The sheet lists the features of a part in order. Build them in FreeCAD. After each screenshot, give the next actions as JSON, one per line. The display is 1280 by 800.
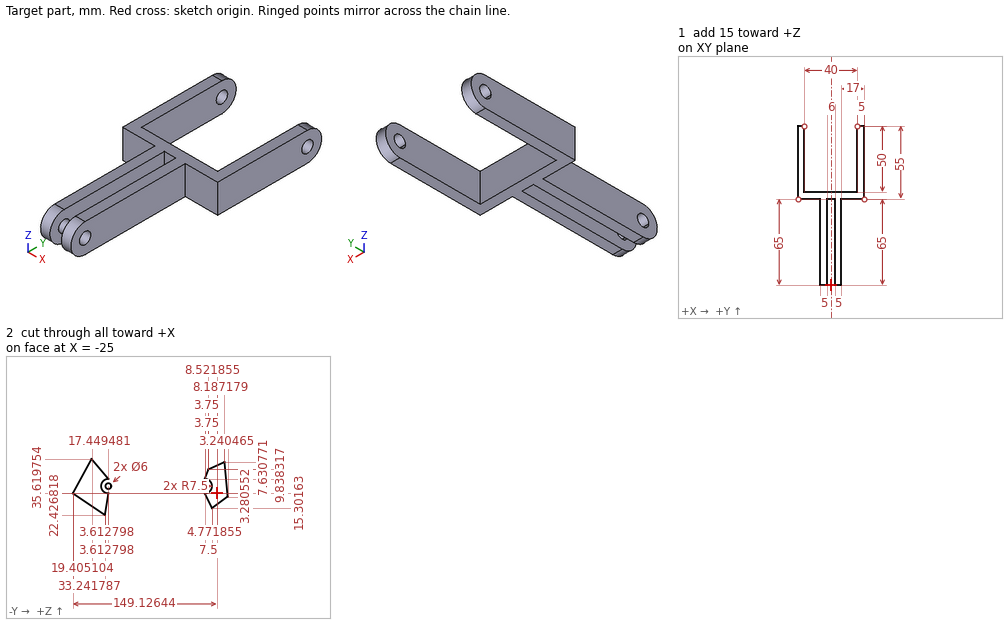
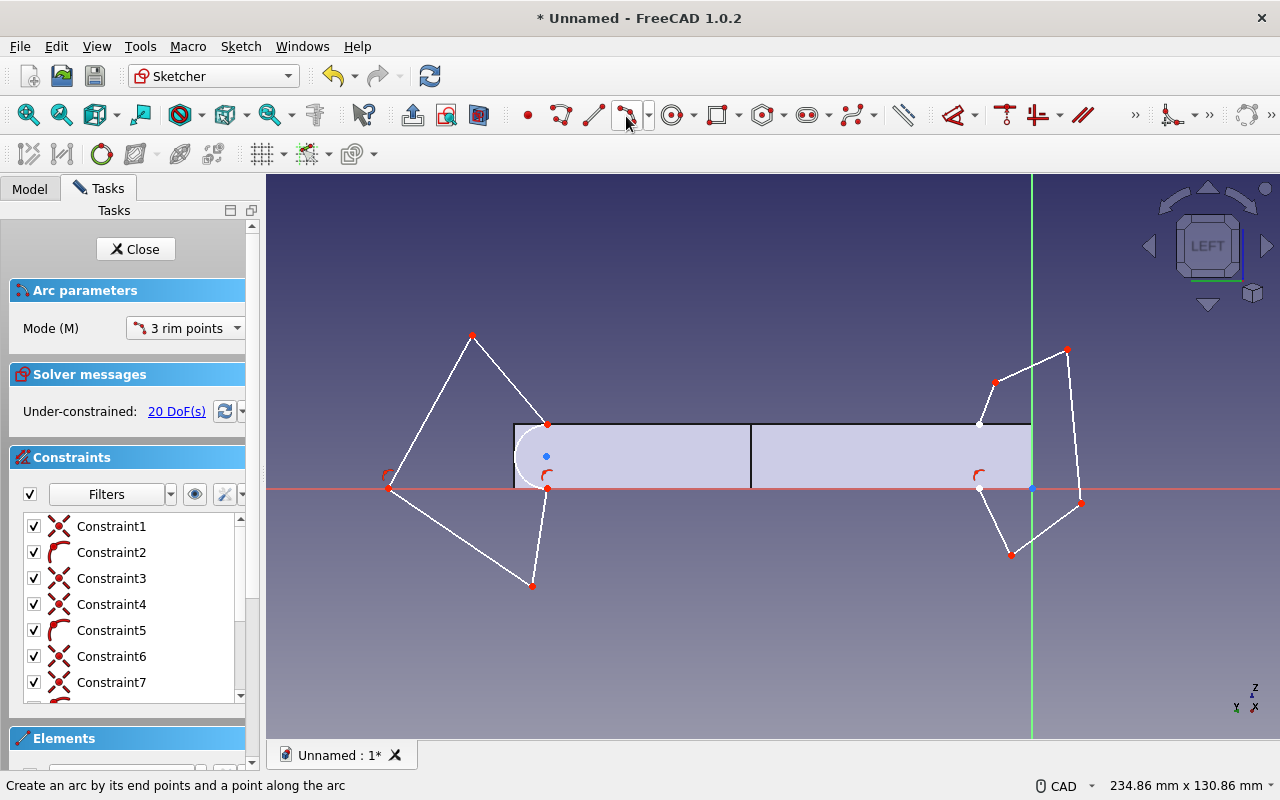
{"action": "left_click", "coordinate": [979, 425]}
{"action": "left_click", "coordinate": [979, 489]}
{"action": "left_click", "coordinate": [1011, 456]}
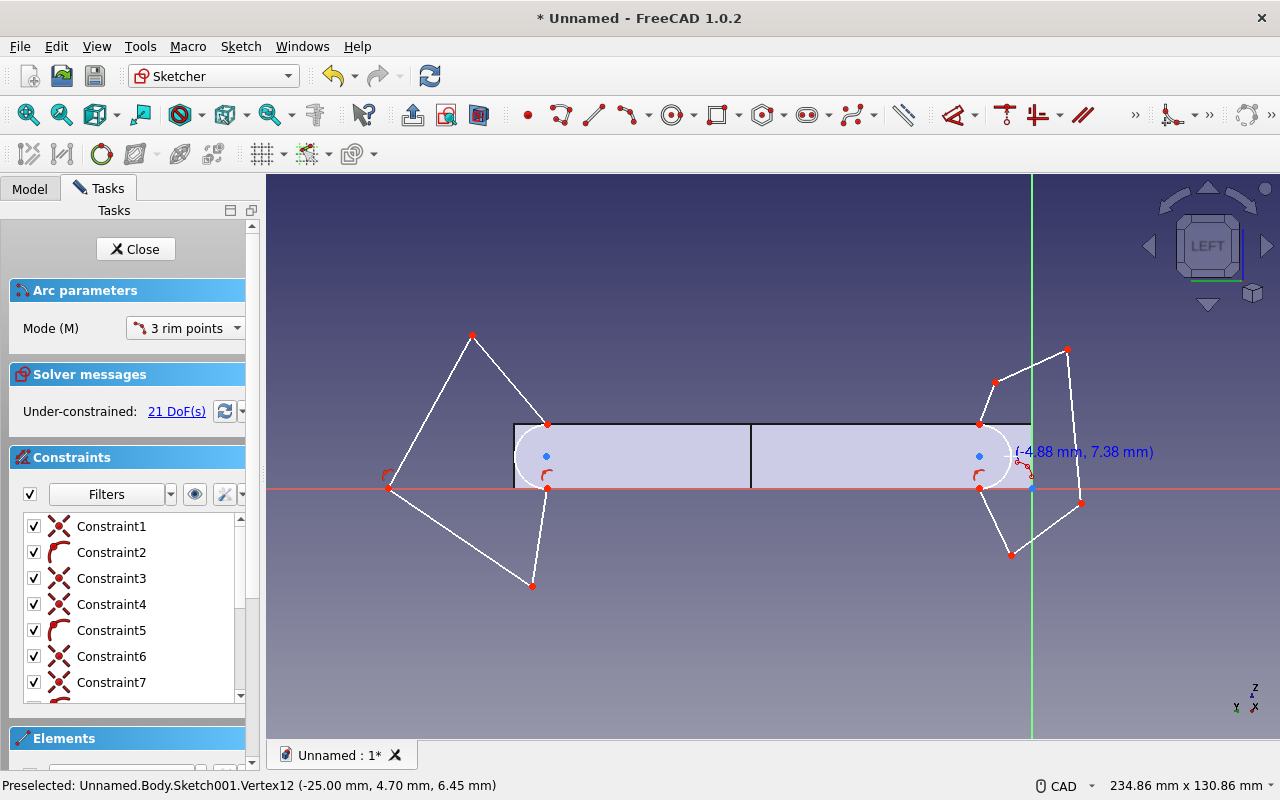
{"action": "key", "text": "g c"}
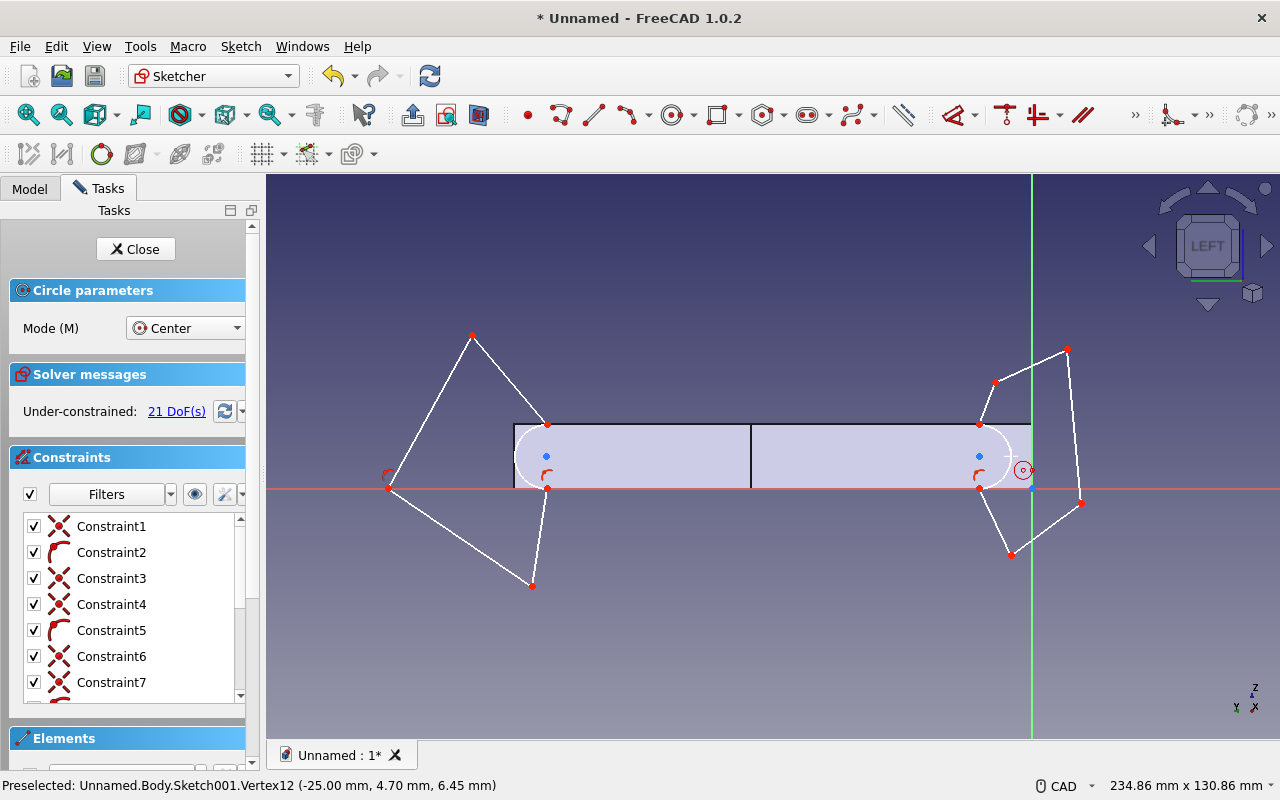
{"action": "scroll", "coordinate": [547, 456], "scroll_direction": "up", "scroll_amount": 3}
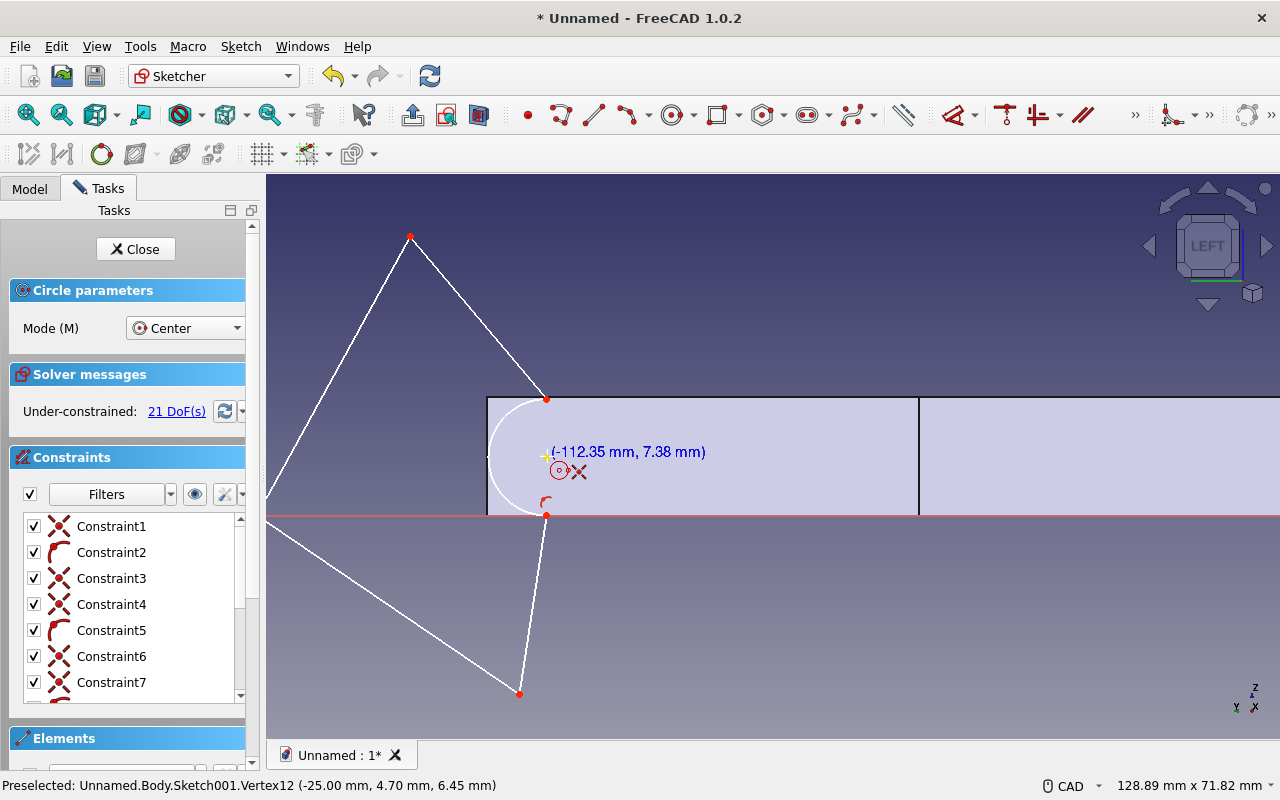
{"action": "left_click", "coordinate": [547, 456]}
{"action": "mouse_move", "coordinate": [564, 440]}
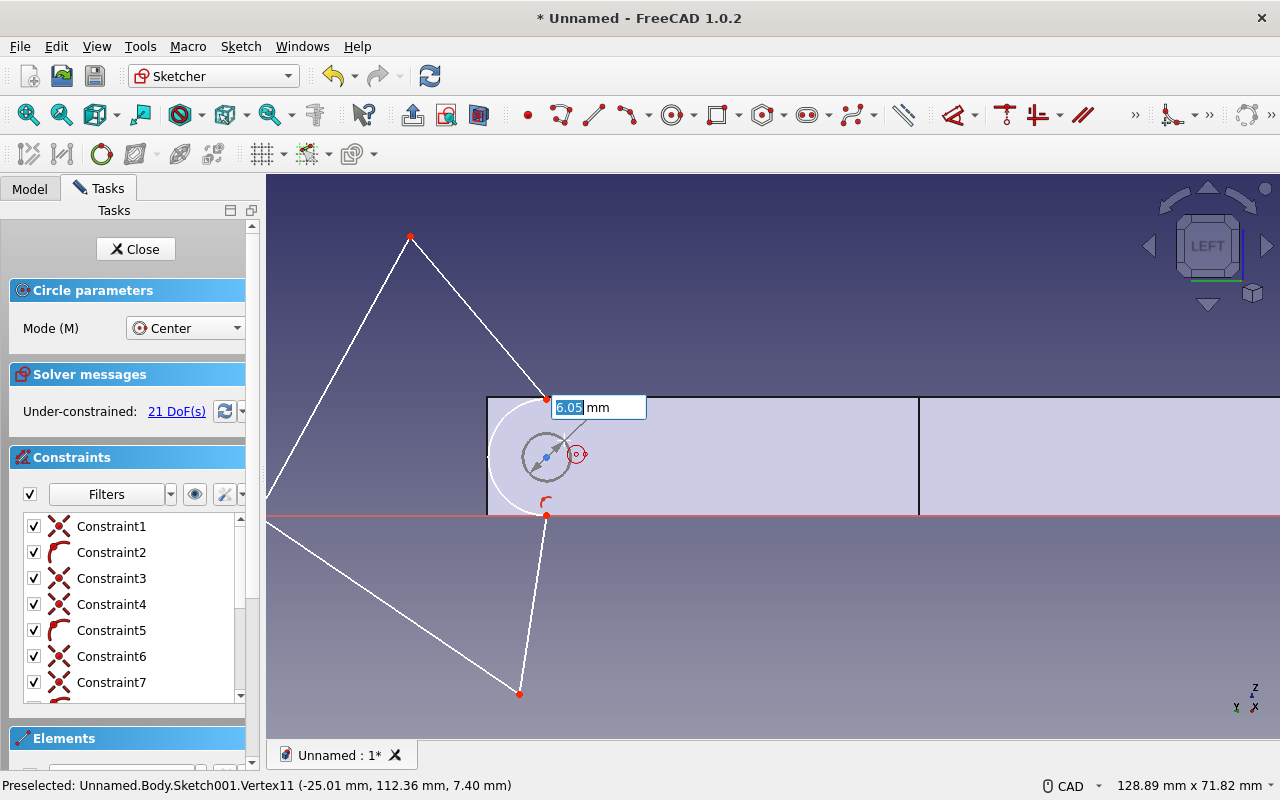
{"action": "type", "text": "6"}
{"action": "key", "text": "Return"}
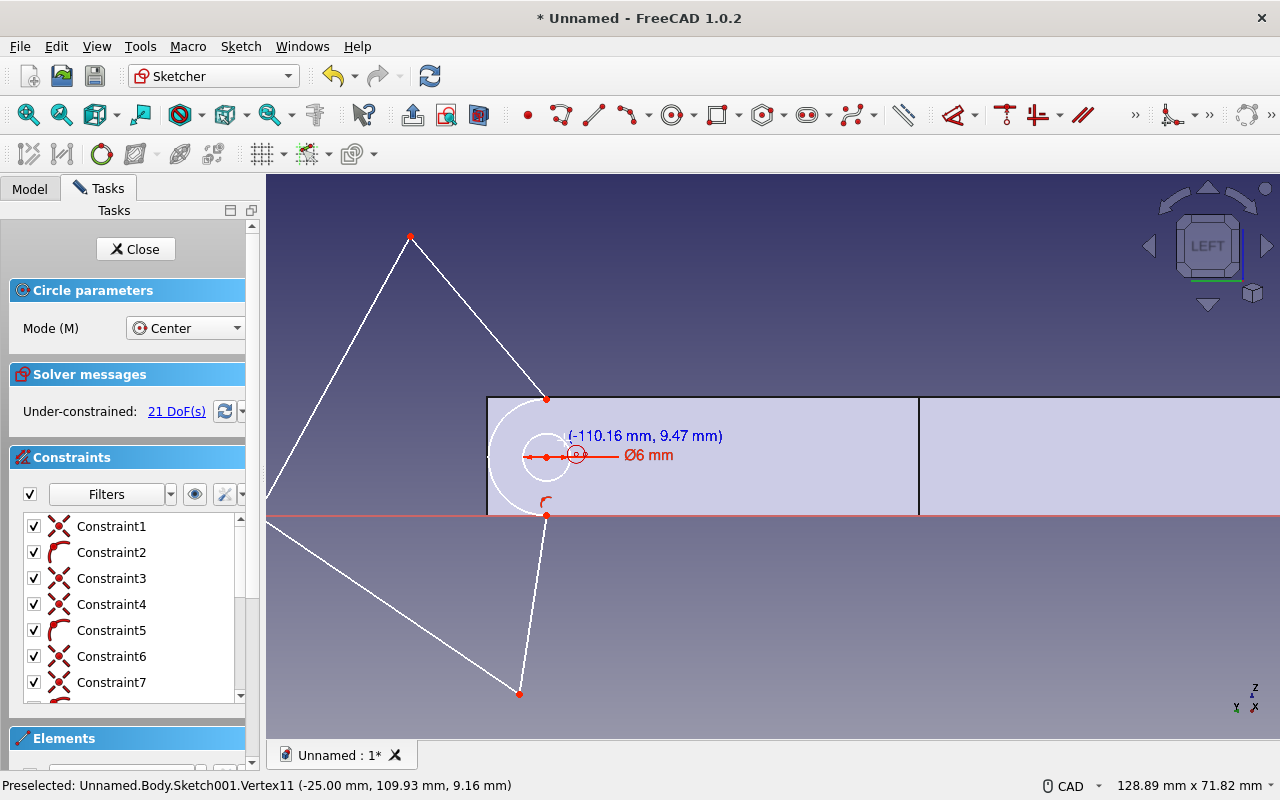
{"action": "scroll", "coordinate": [554, 451], "scroll_direction": "down", "scroll_amount": 4}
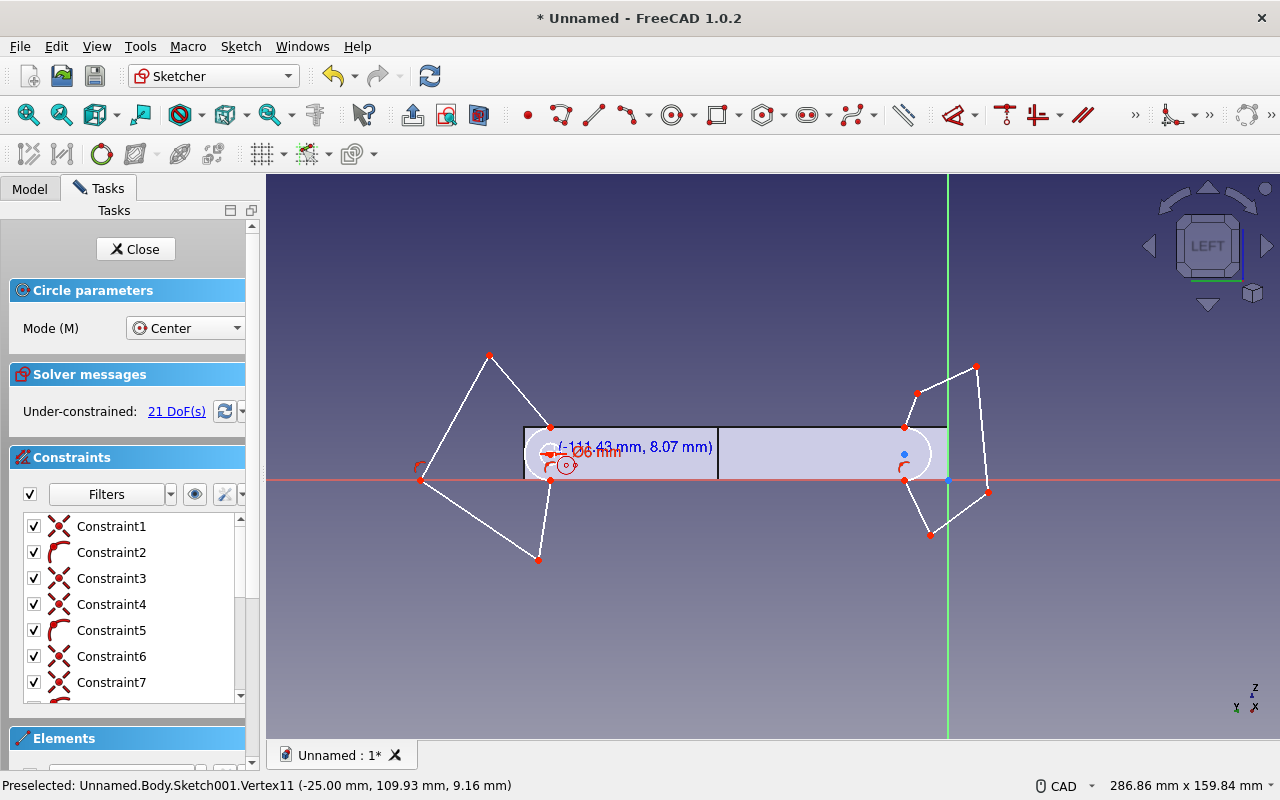
{"action": "scroll", "coordinate": [905, 454], "scroll_direction": "up", "scroll_amount": 4}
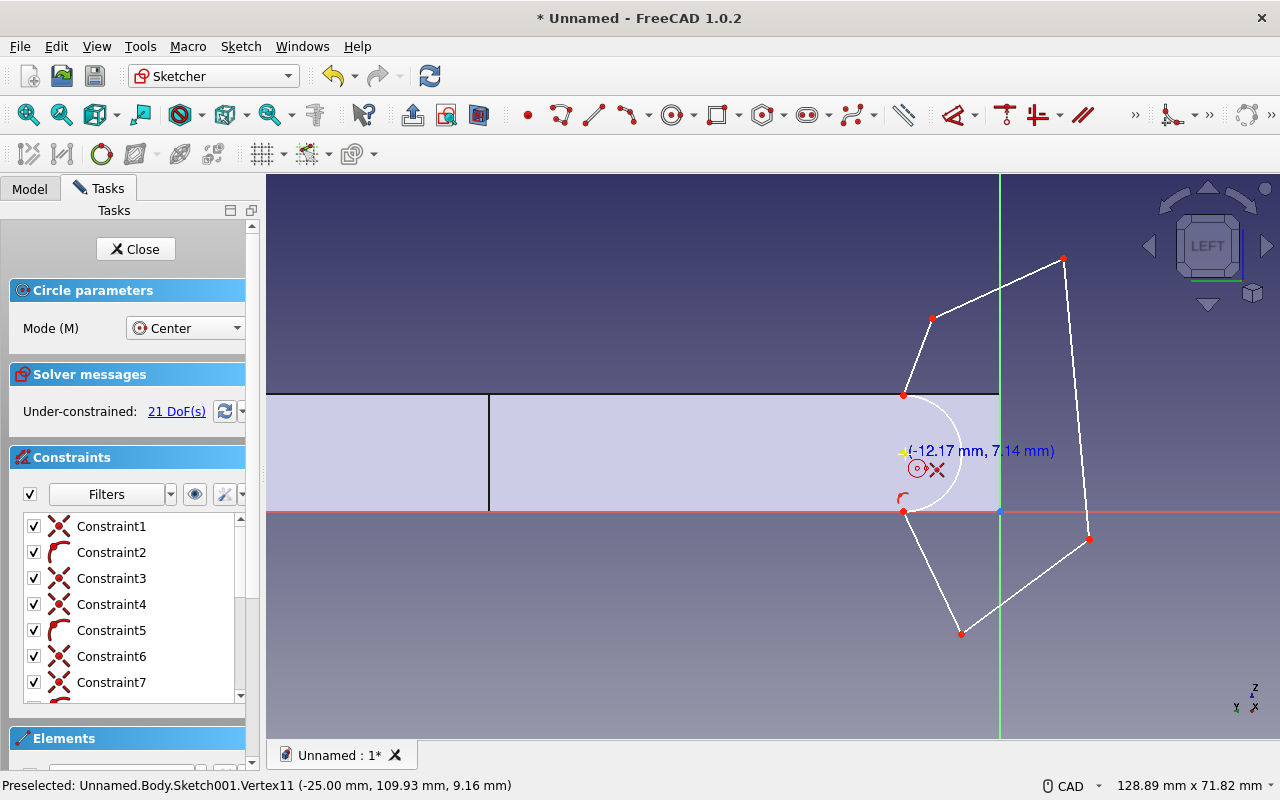
{"action": "left_click", "coordinate": [903, 453]}
{"action": "mouse_move", "coordinate": [920, 436]}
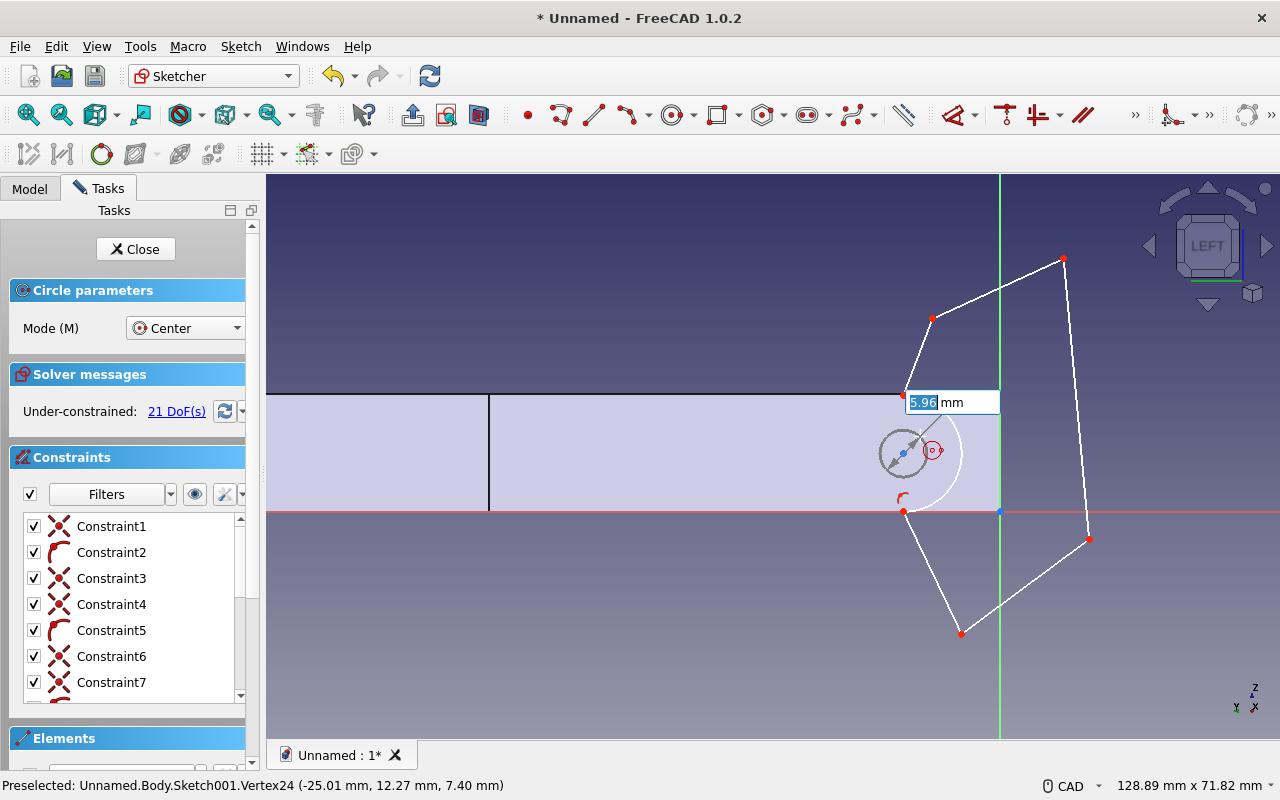
{"action": "type", "text": "6"}
{"action": "key", "text": "Return"}
{"action": "key", "text": "Escape"}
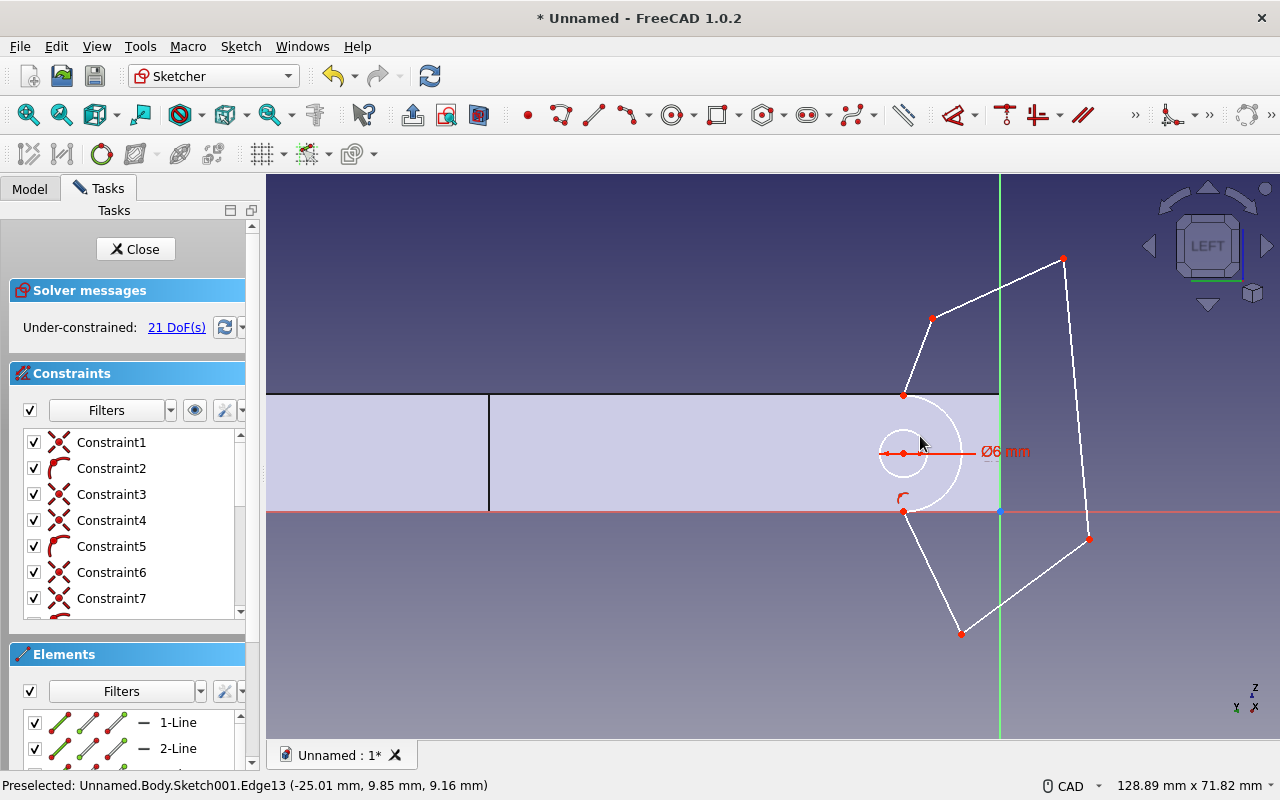
{"action": "scroll", "coordinate": [905, 454], "scroll_direction": "down", "scroll_amount": 4}